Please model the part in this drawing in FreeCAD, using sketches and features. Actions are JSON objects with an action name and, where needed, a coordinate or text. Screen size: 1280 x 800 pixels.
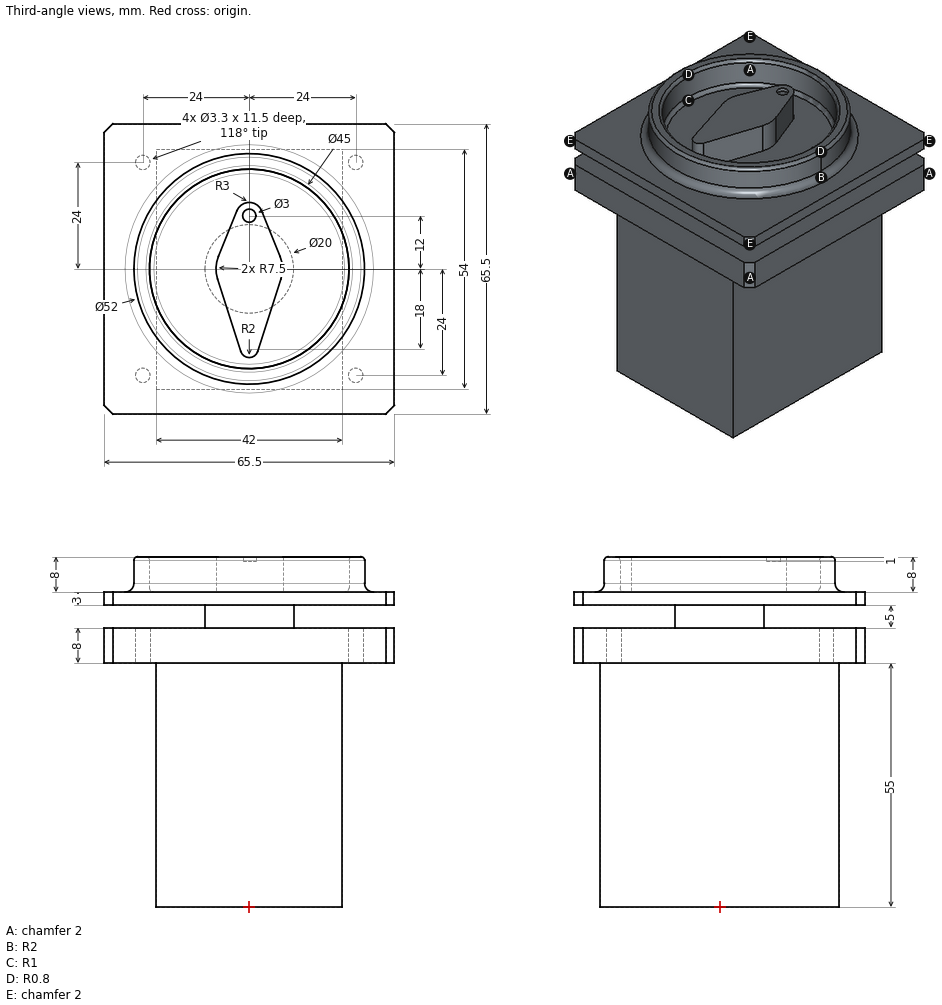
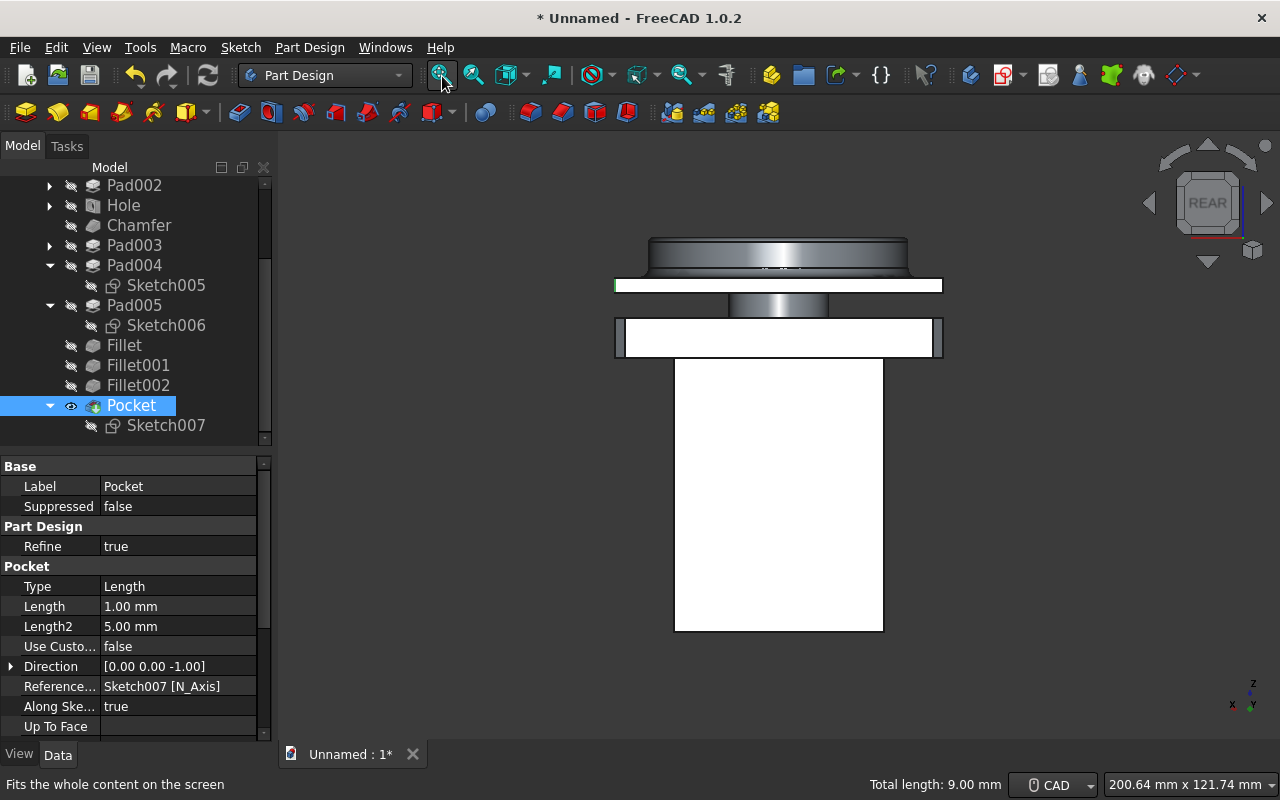
{"action": "left_click", "coordinate": [943, 284], "text": "ctrl"}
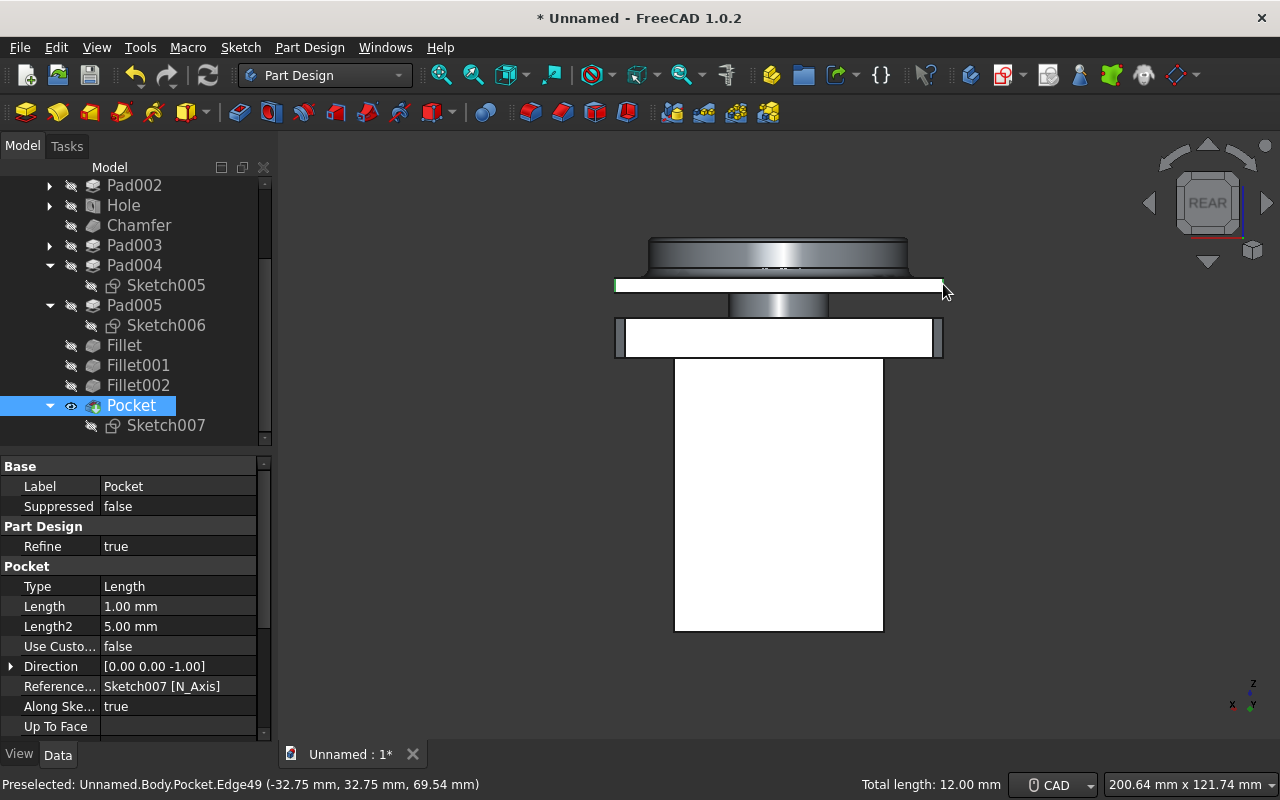
{"action": "left_click", "coordinate": [564, 112]}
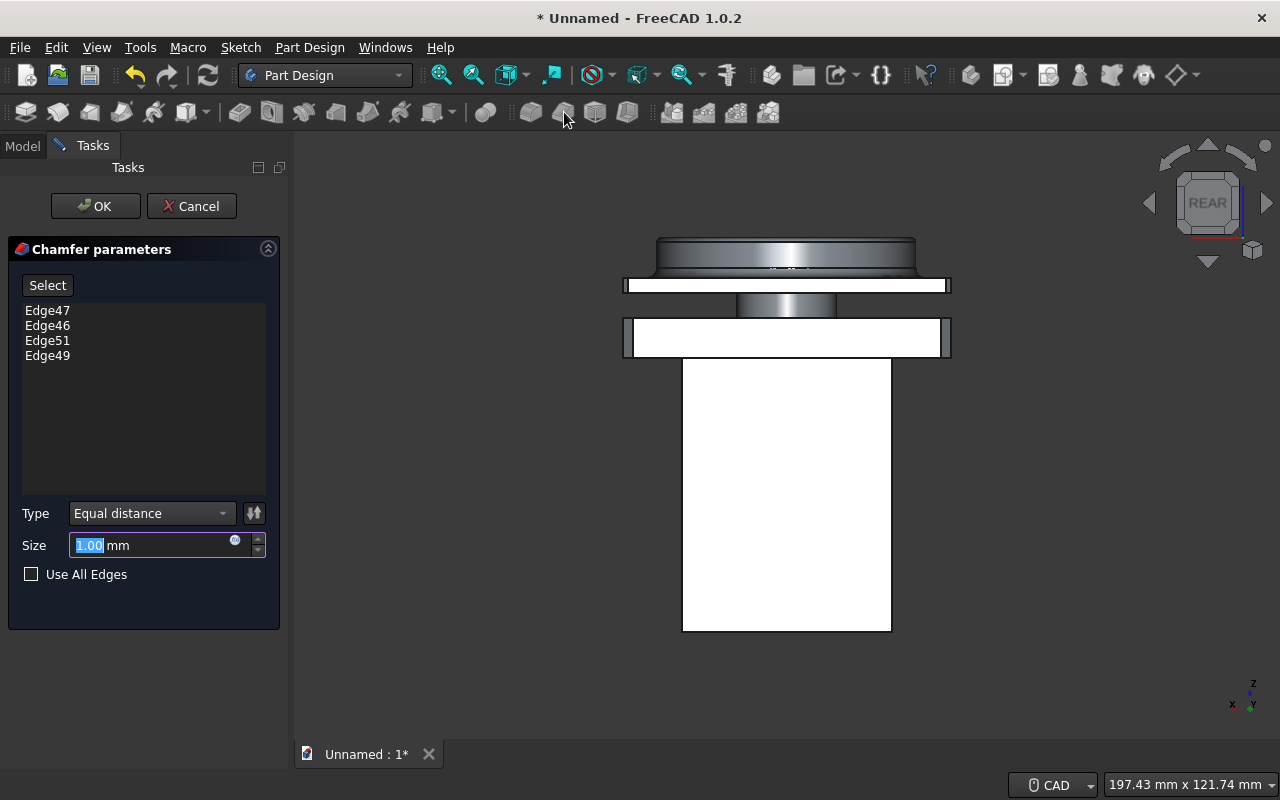
{"action": "type", "text": "2"}
{"action": "key", "text": "Tab"}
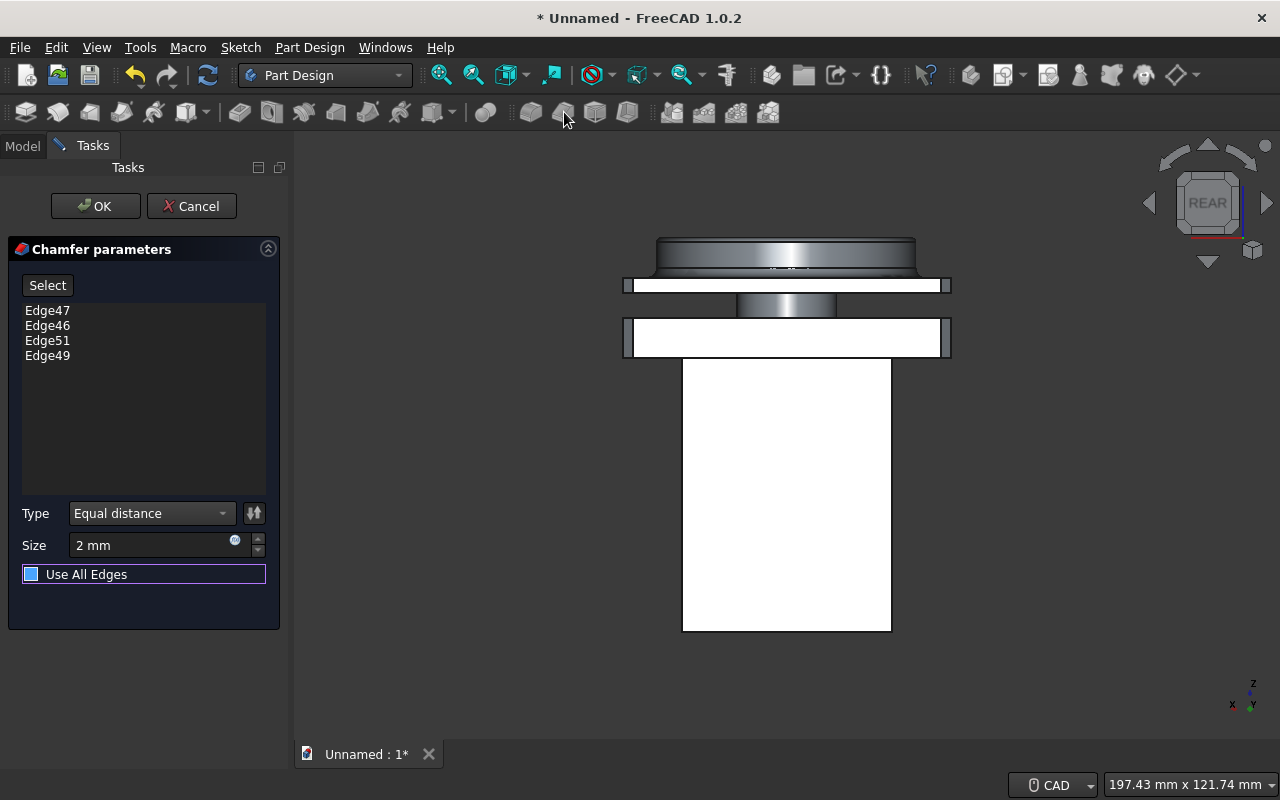
{"action": "left_click", "coordinate": [96, 206]}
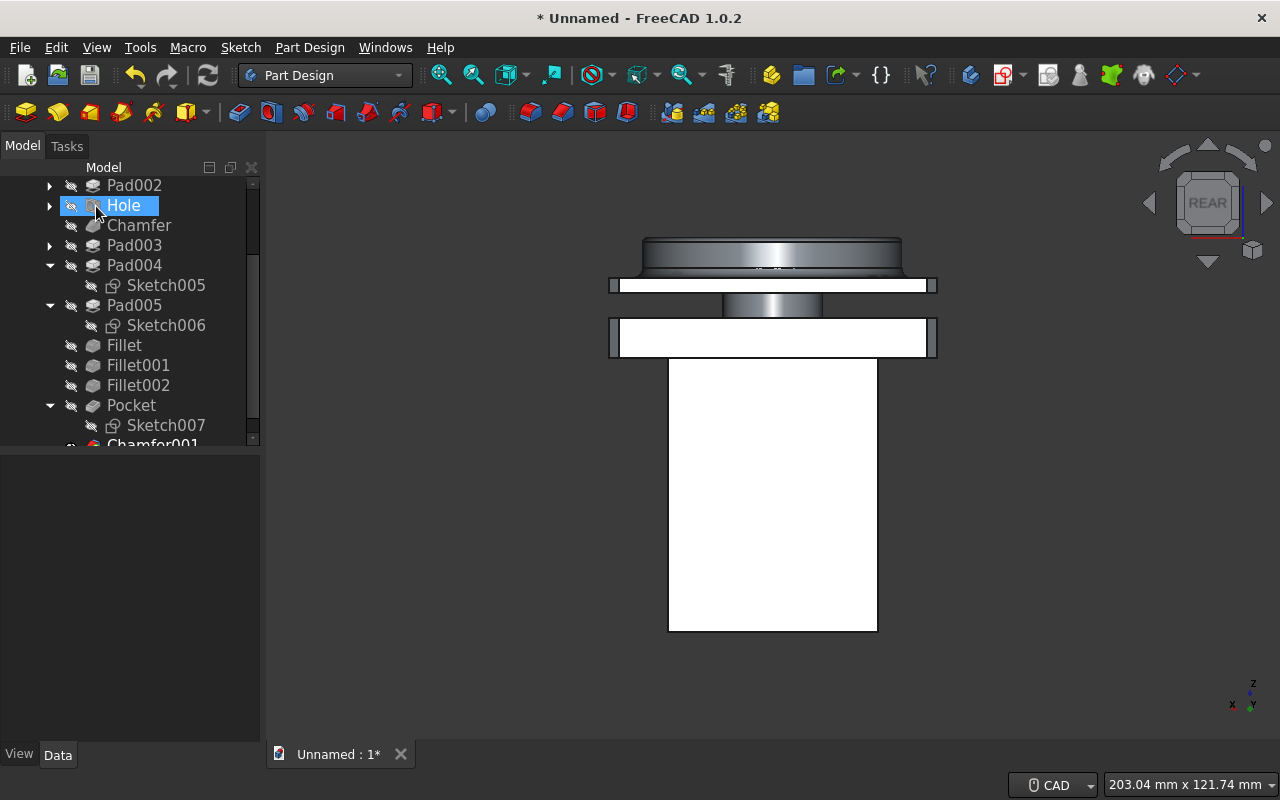
{"action": "key", "text": "0"}